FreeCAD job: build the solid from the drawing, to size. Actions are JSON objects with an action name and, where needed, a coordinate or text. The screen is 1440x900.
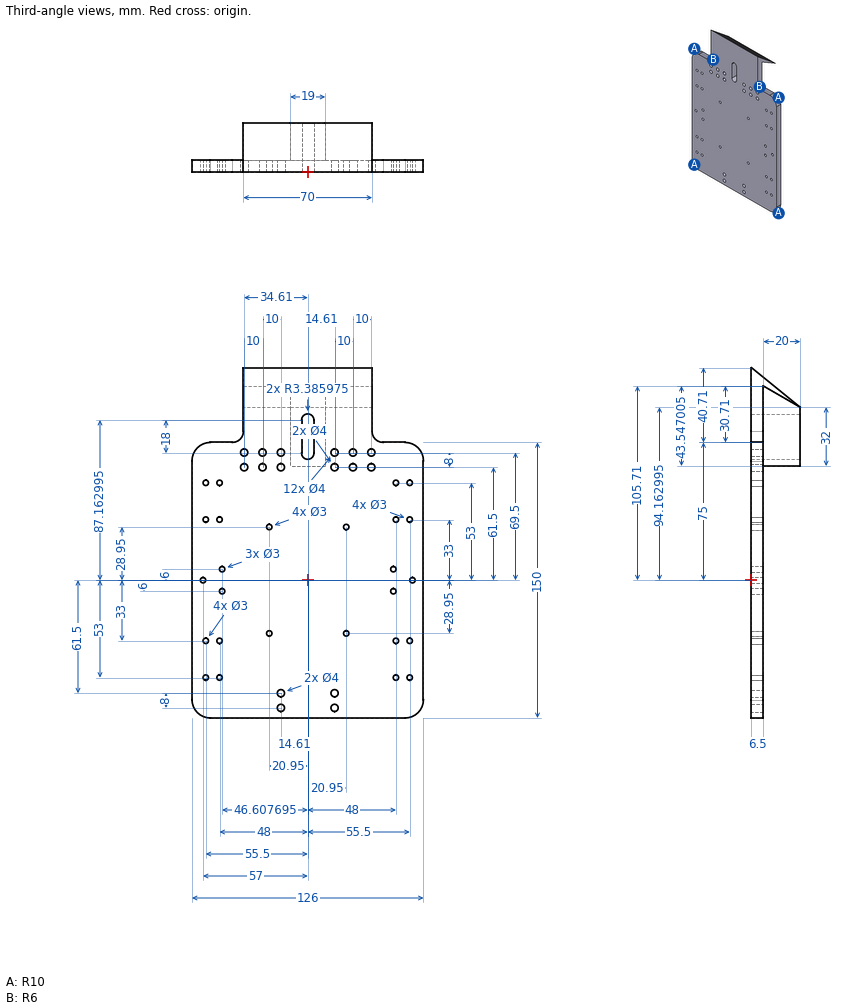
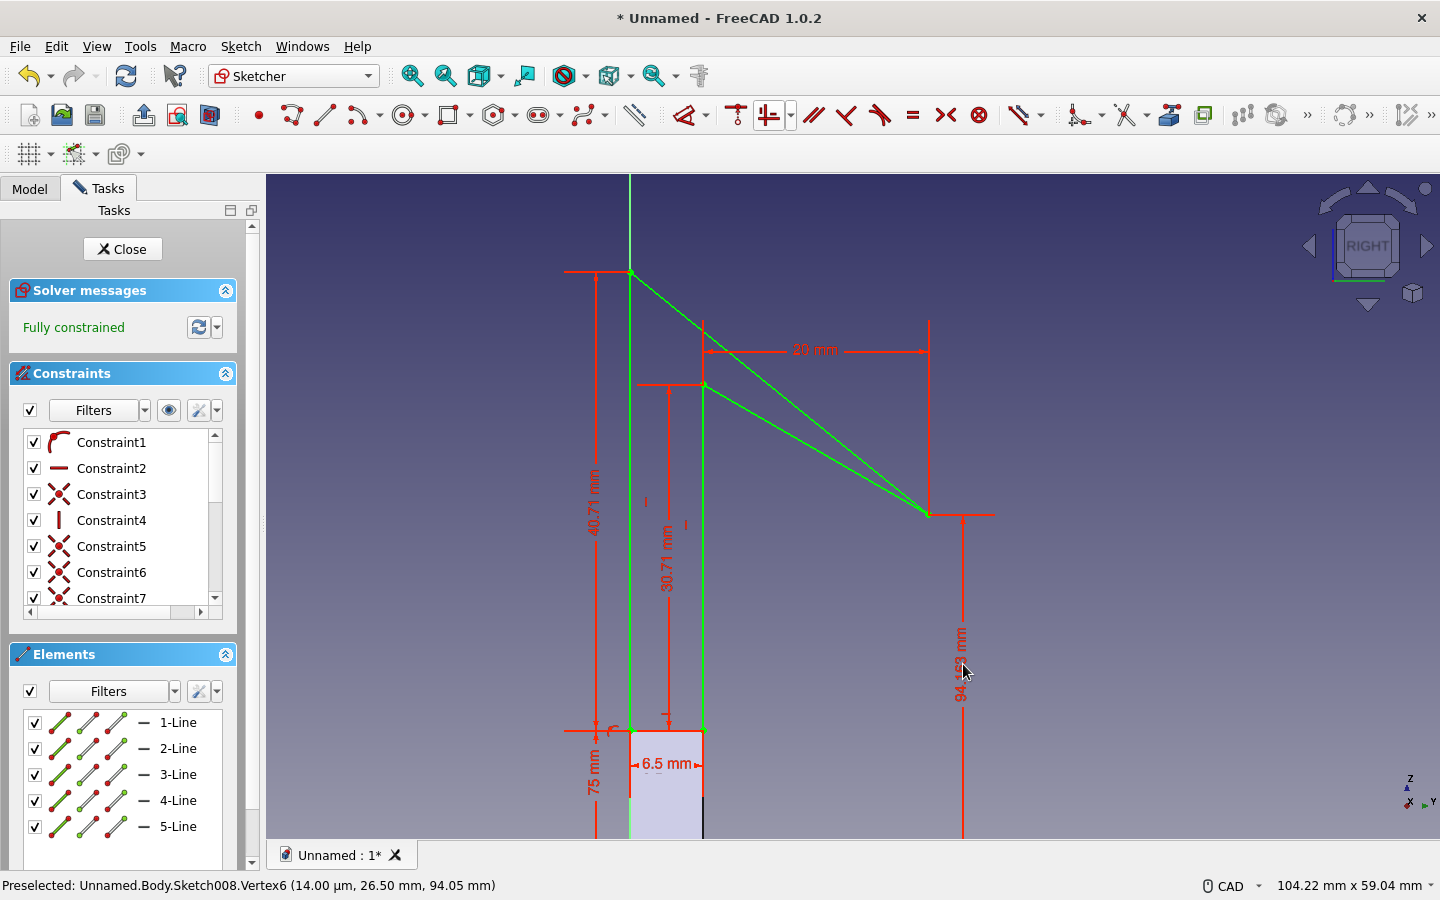
{"action": "left_click", "coordinate": [123, 249]}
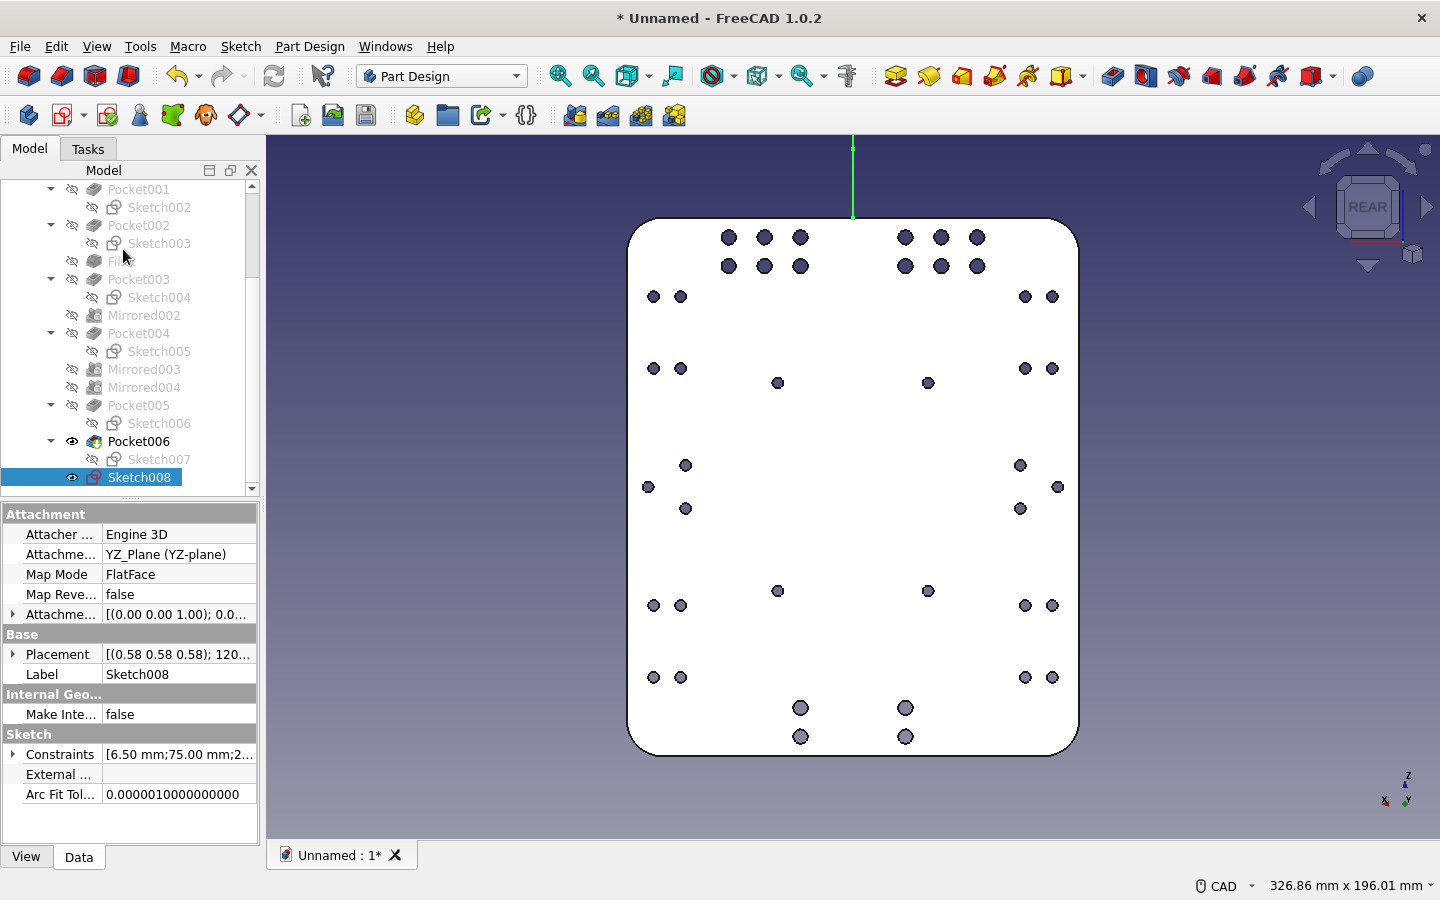
{"action": "left_click", "coordinate": [896, 76]}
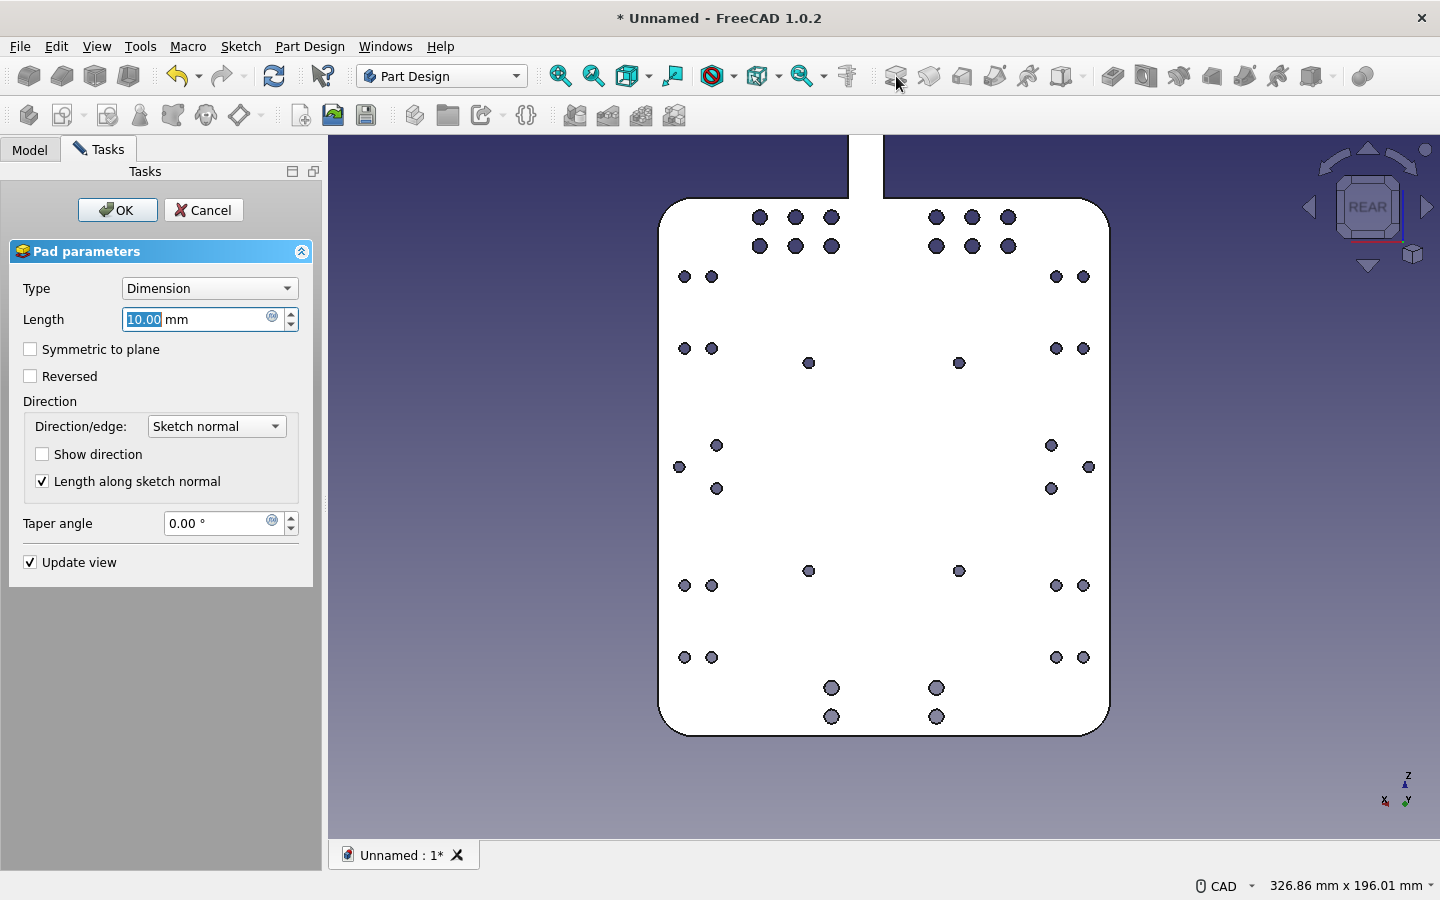
{"action": "type", "text": "70"}
{"action": "key", "text": "Tab"}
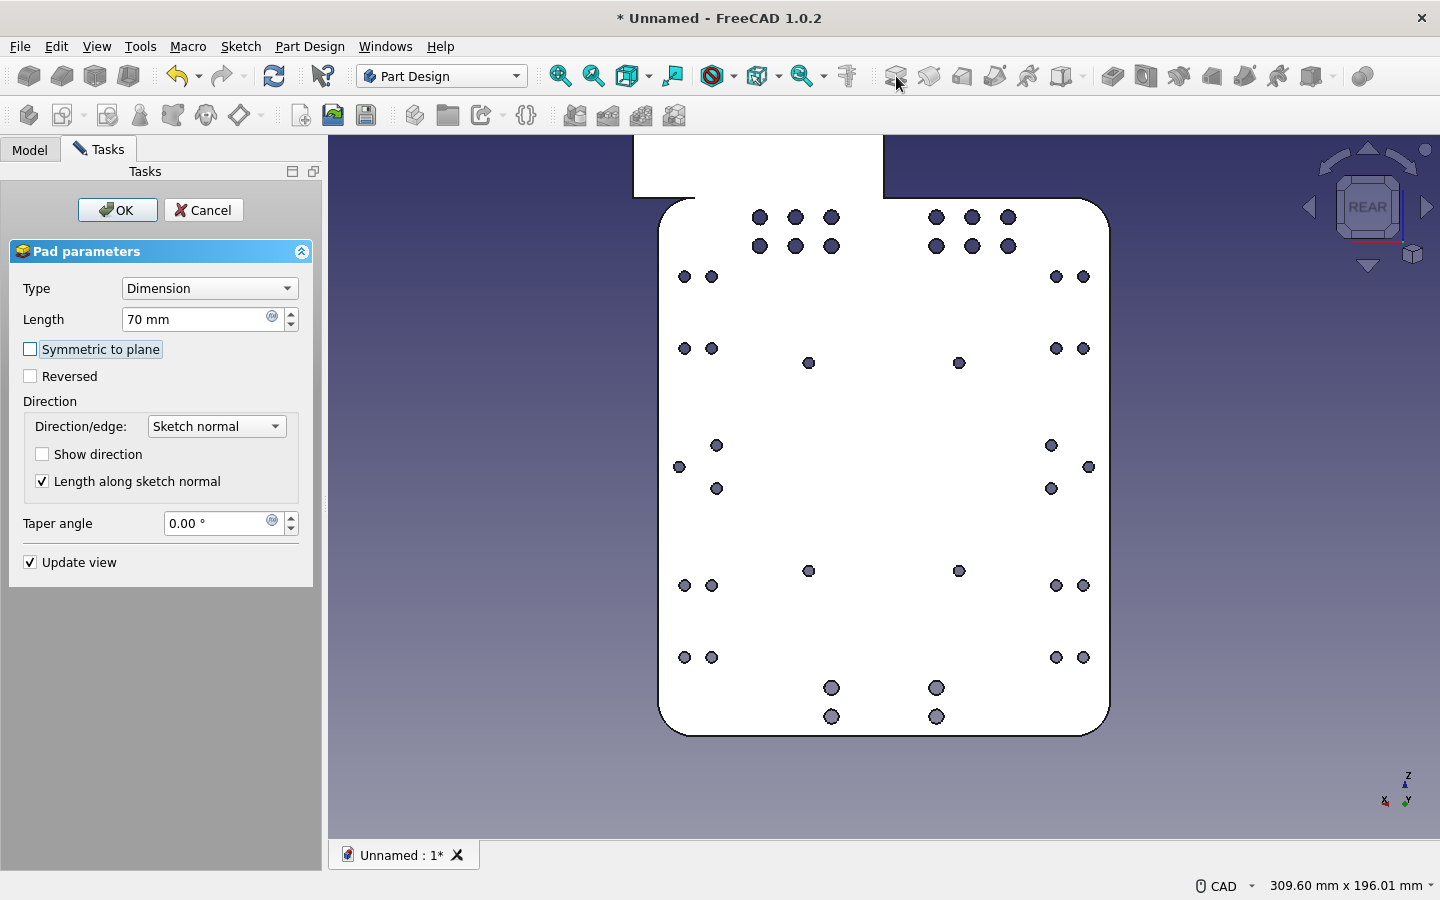
{"action": "left_click", "coordinate": [31, 349]}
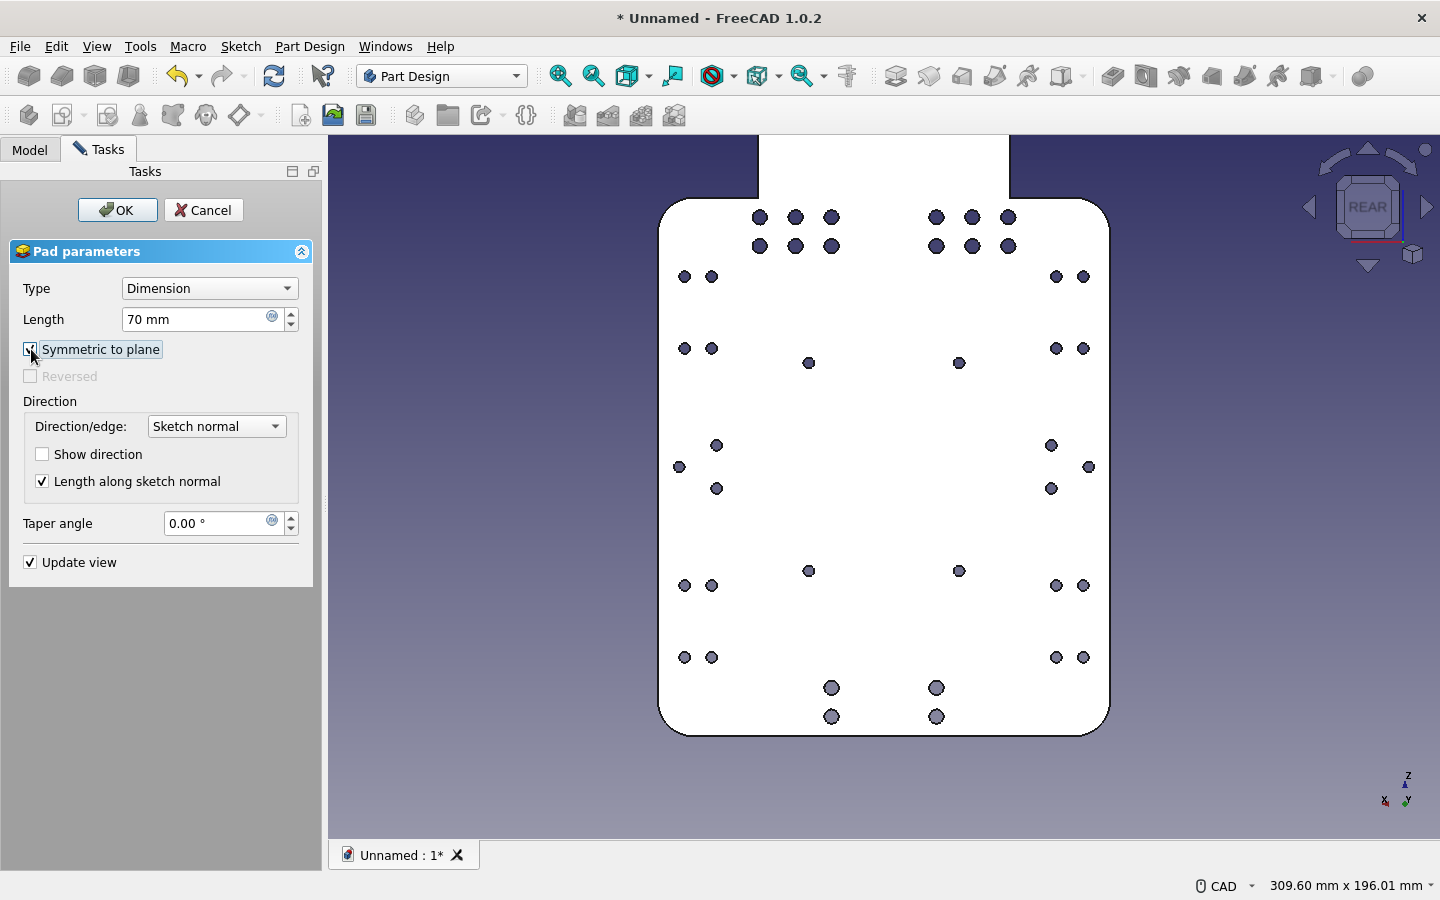
{"action": "left_click", "coordinate": [118, 210]}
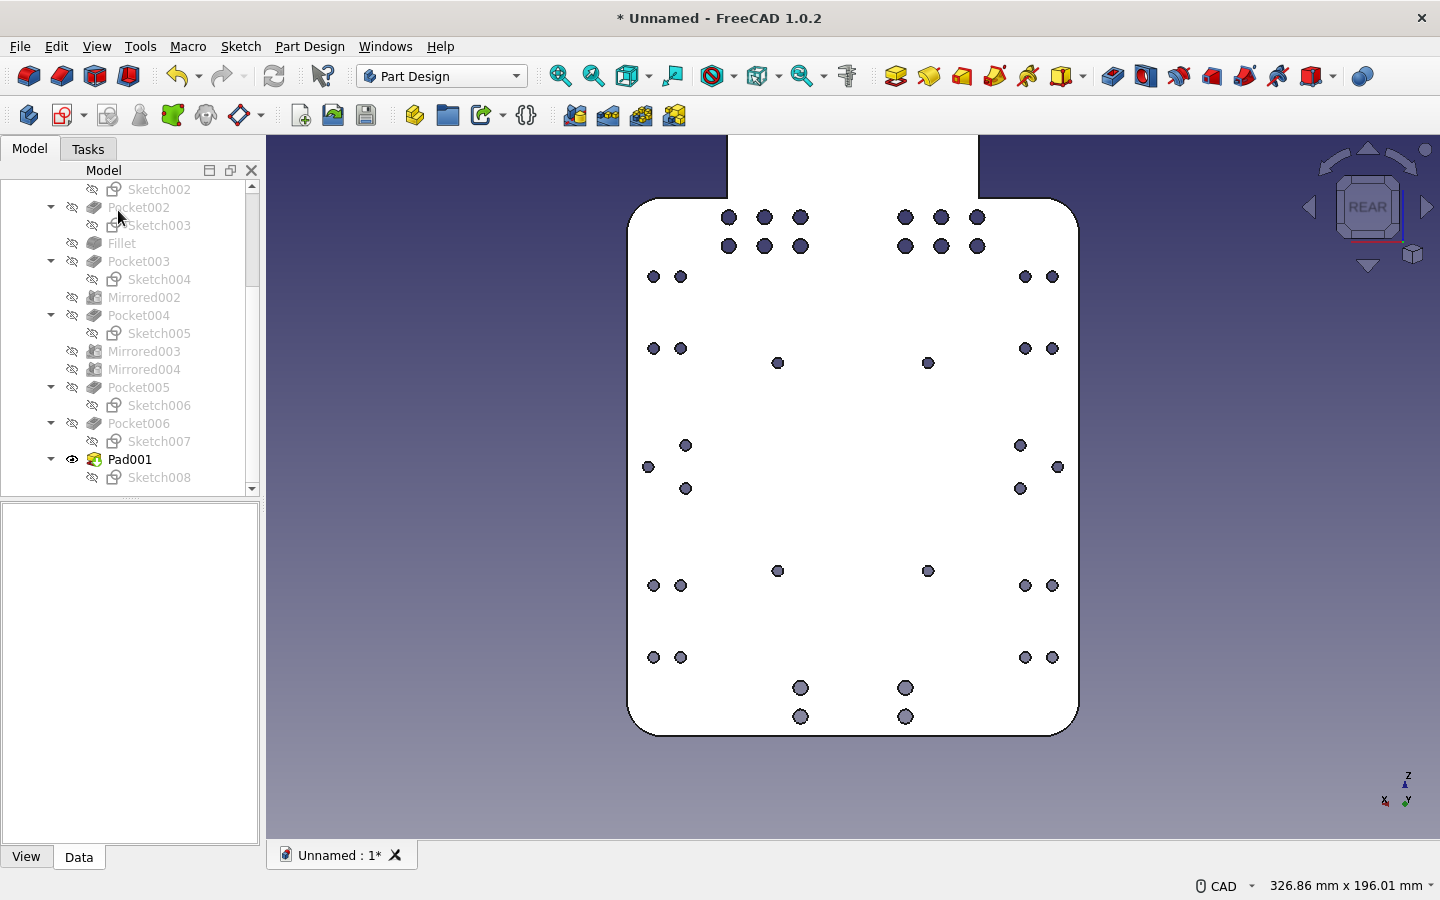
{"action": "left_click", "coordinate": [561, 76]}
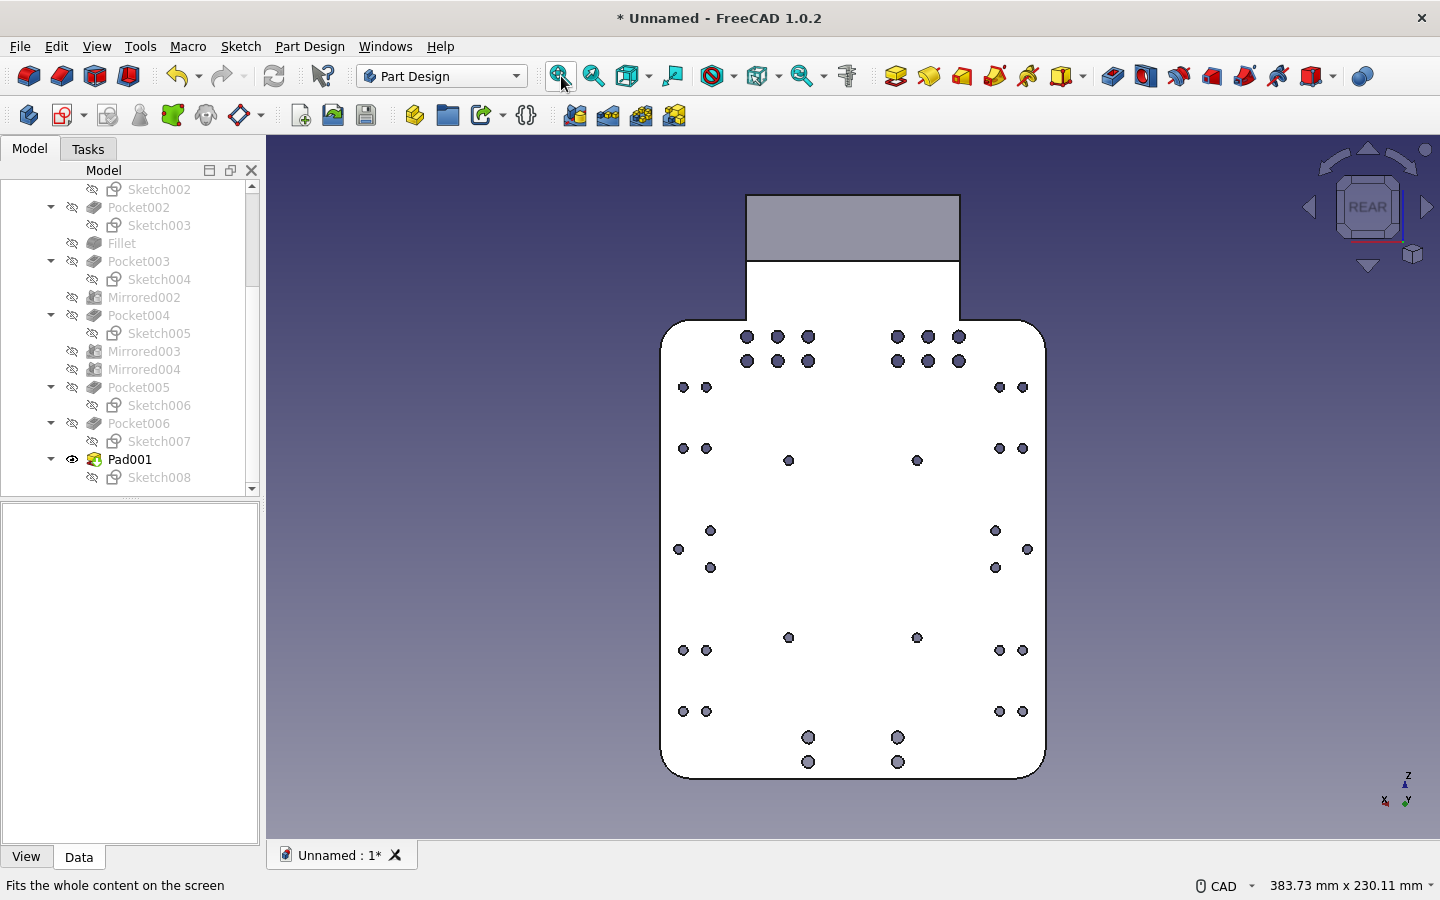
{"action": "left_click", "coordinate": [62, 116]}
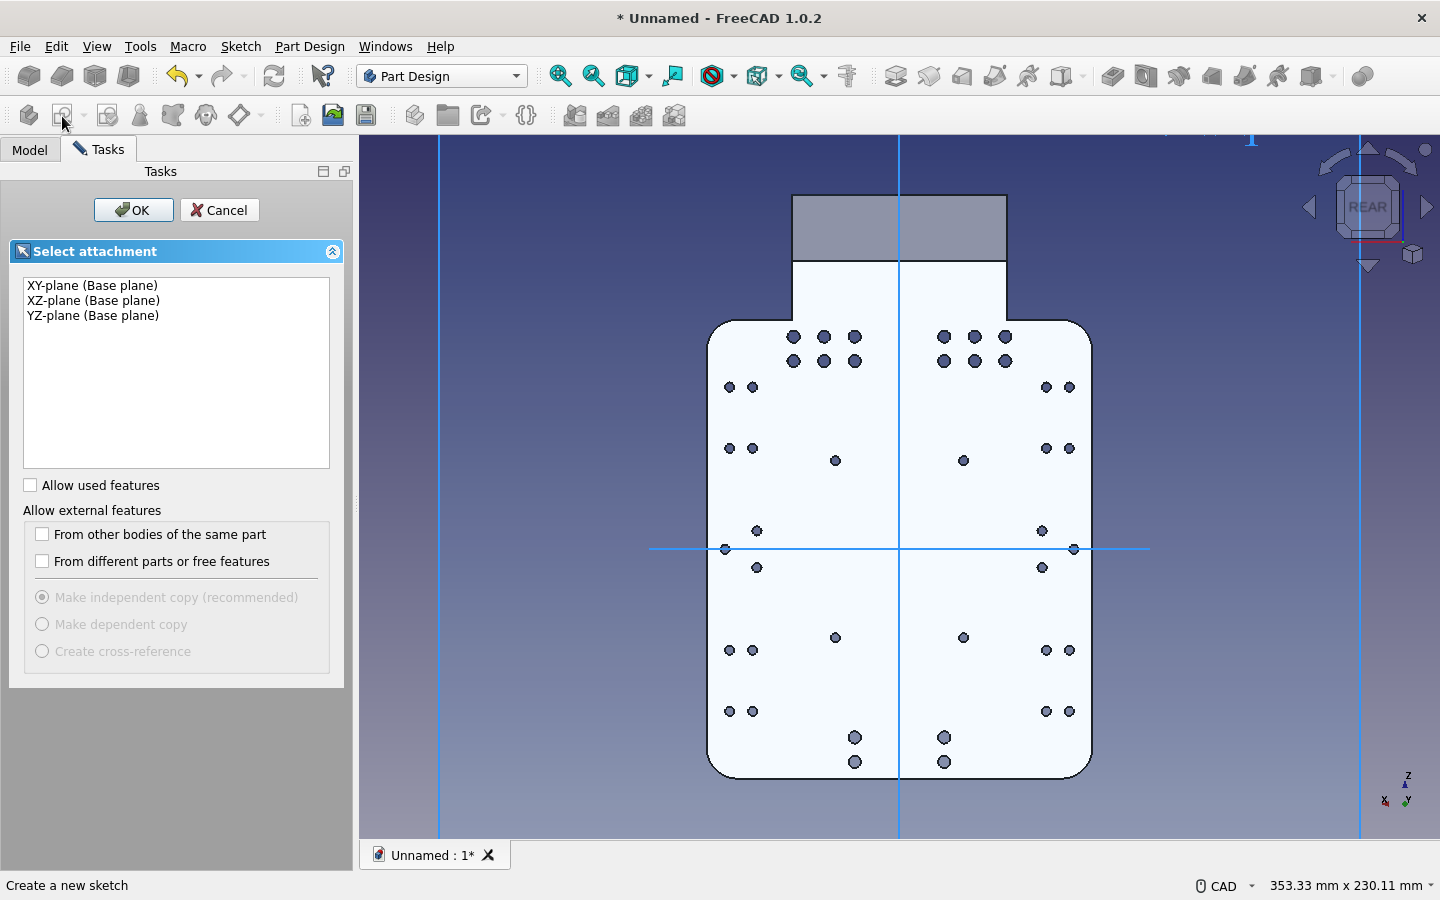
{"action": "left_click", "coordinate": [84, 316]}